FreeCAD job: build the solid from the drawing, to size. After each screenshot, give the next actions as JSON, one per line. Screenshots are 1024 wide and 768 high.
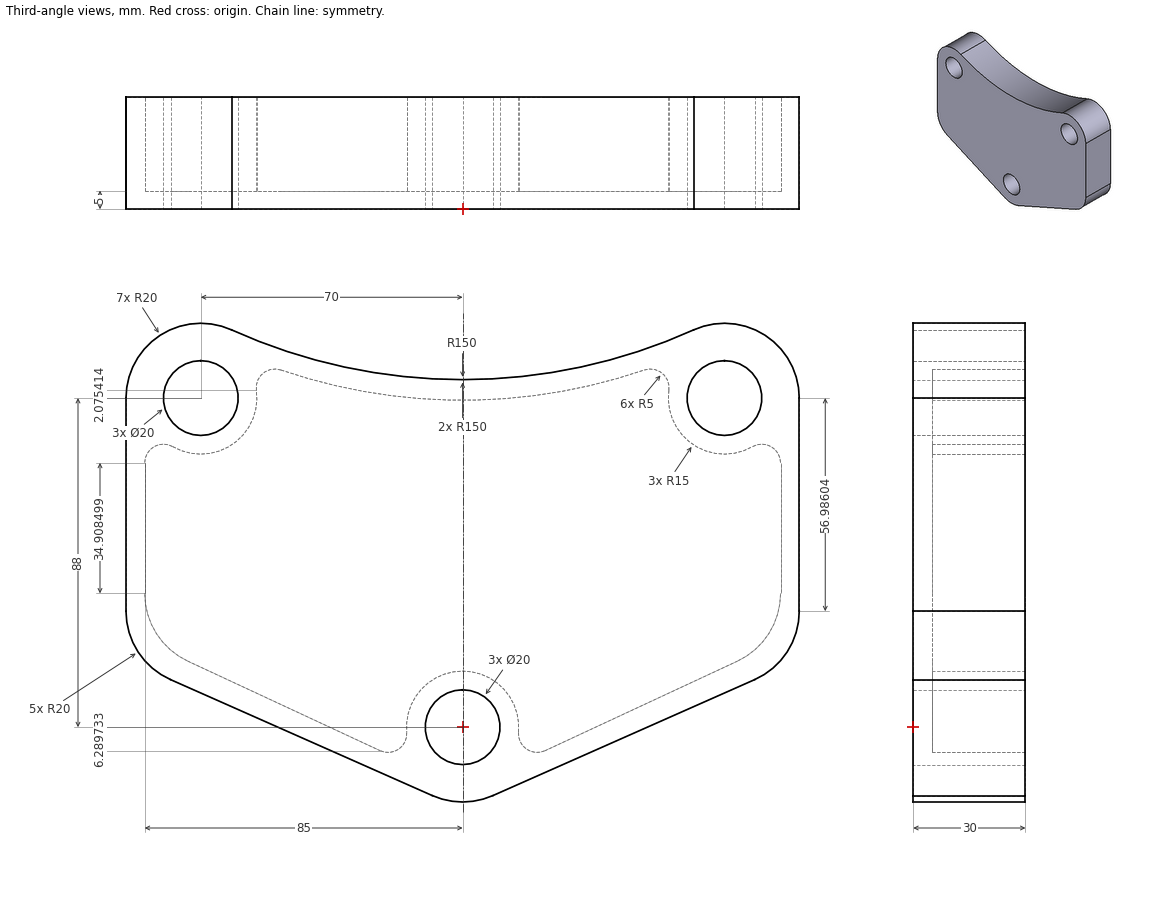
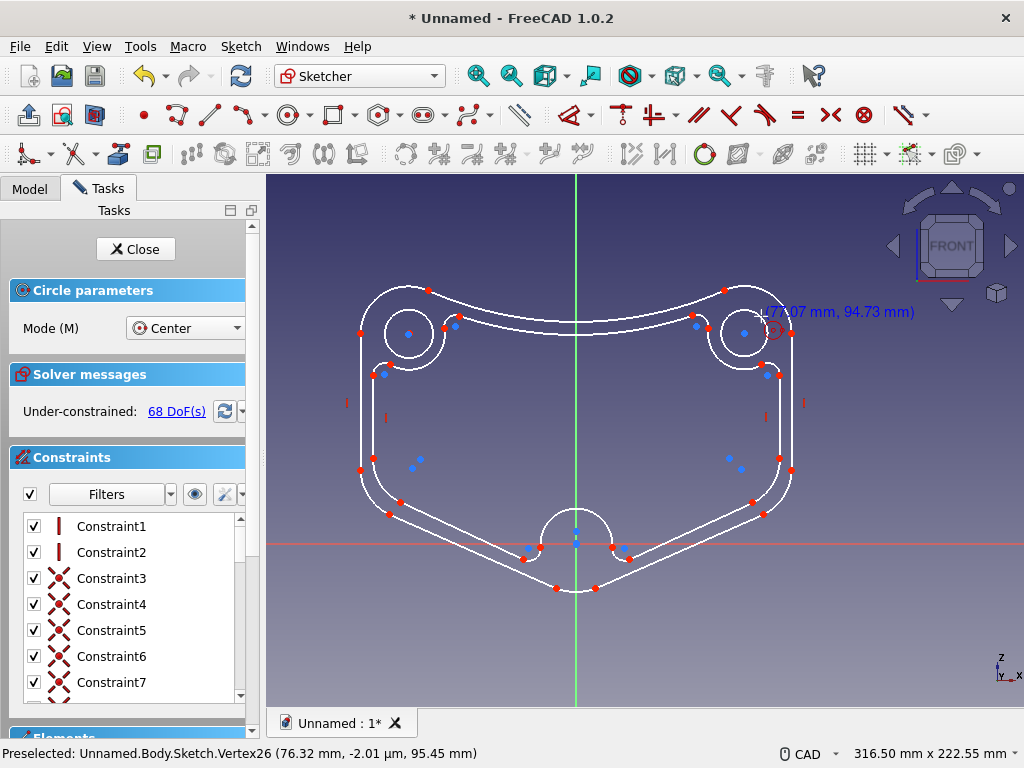
{"action": "left_click", "coordinate": [576, 544]}
{"action": "left_click", "coordinate": [593, 561]}
{"action": "key", "text": "Escape"}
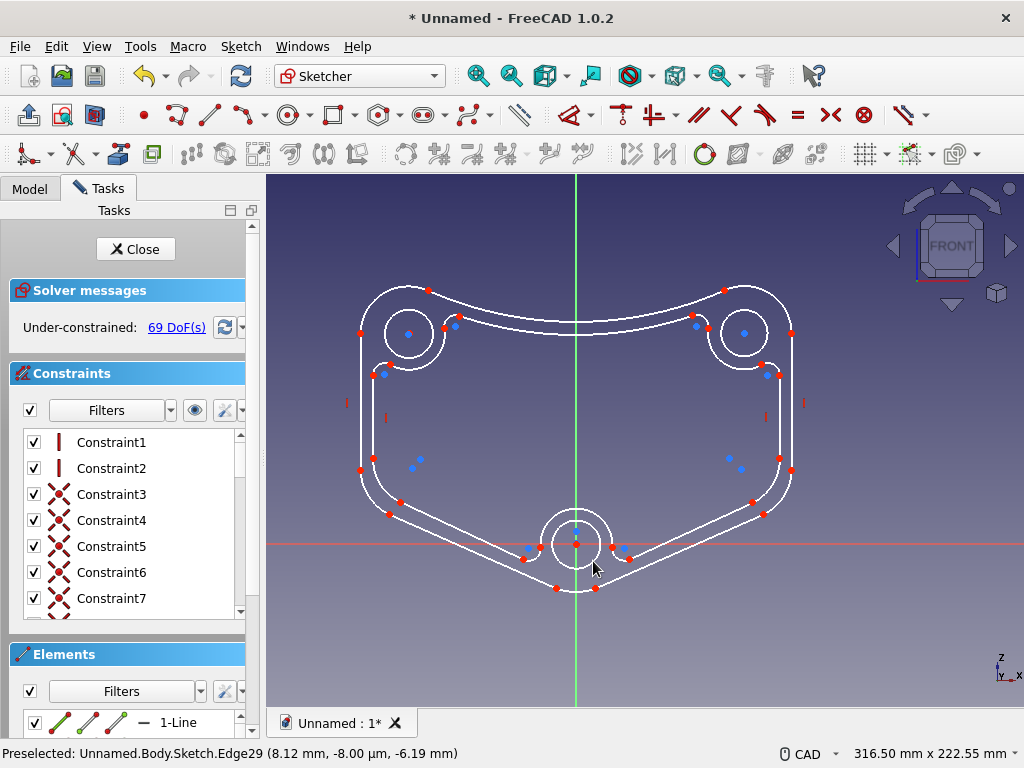
{"action": "left_click", "coordinate": [792, 375]}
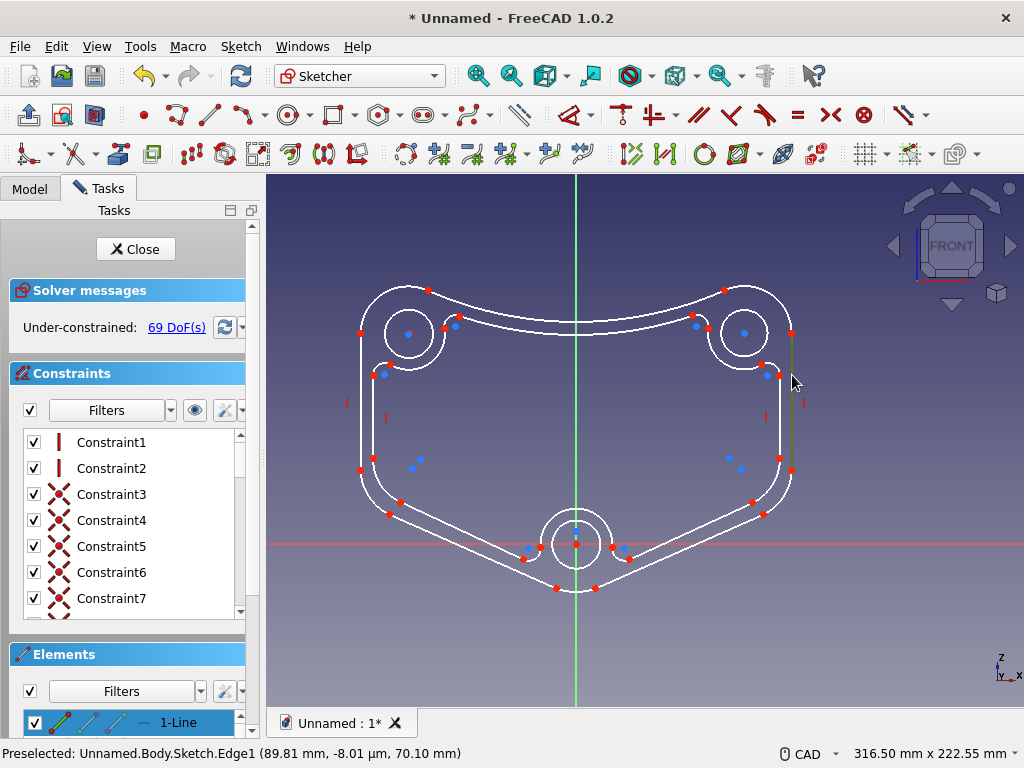
{"action": "left_click", "coordinate": [777, 505]}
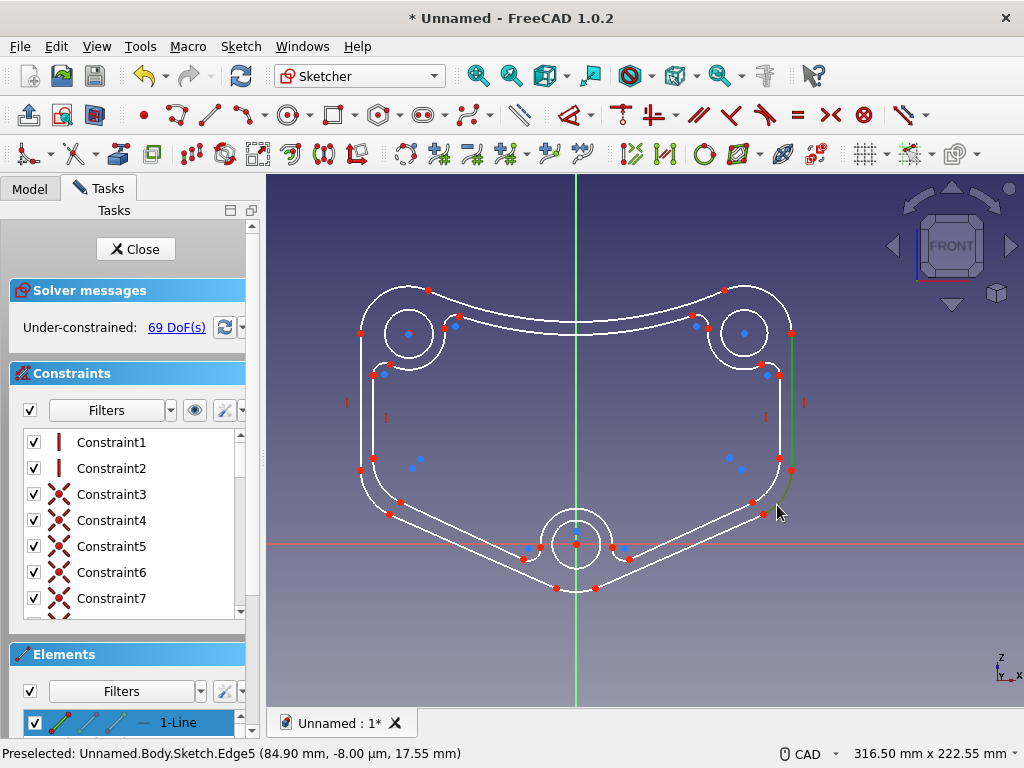
{"action": "key", "text": "t"}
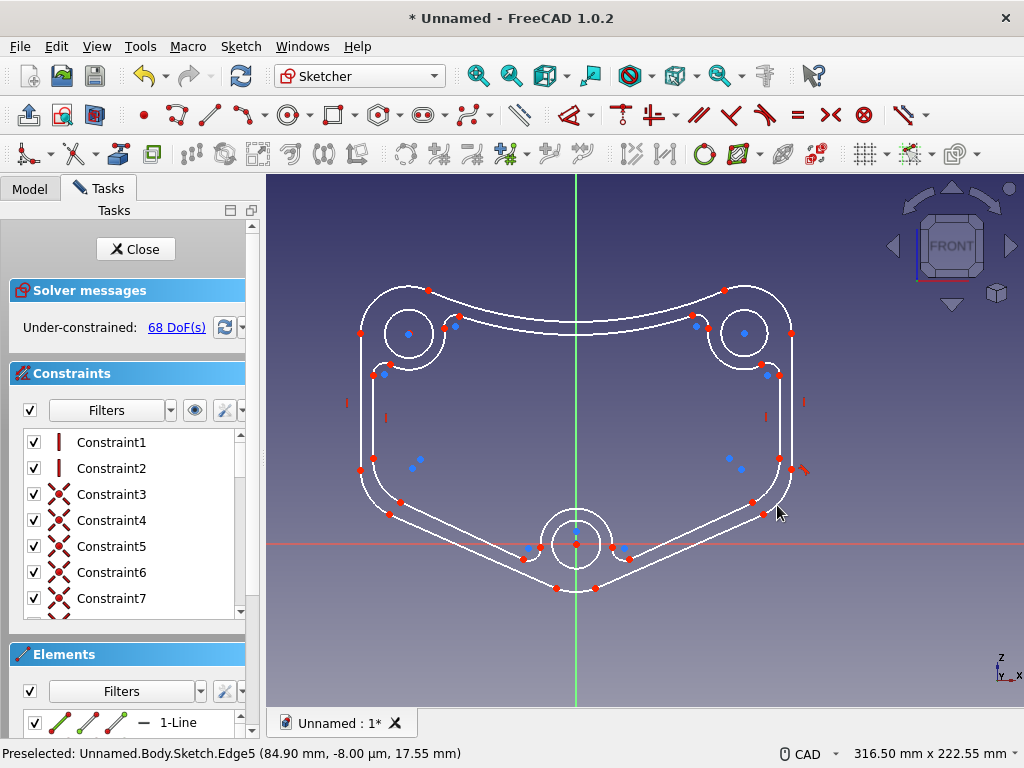
{"action": "left_click", "coordinate": [792, 374]}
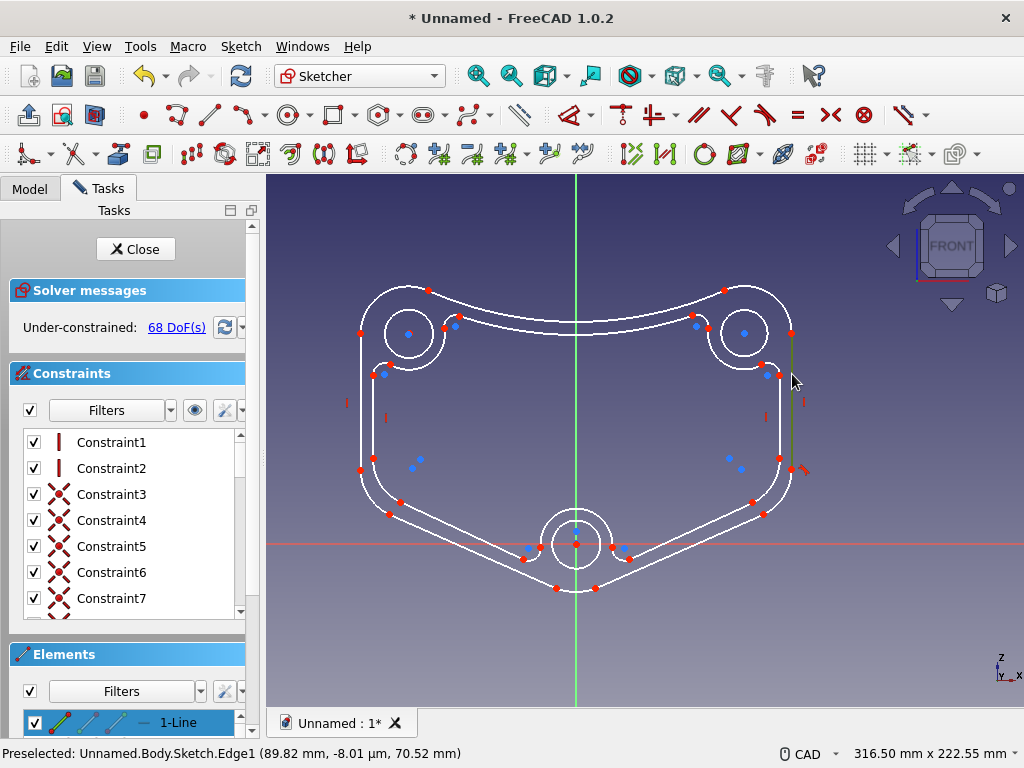
{"action": "left_click", "coordinate": [783, 307]}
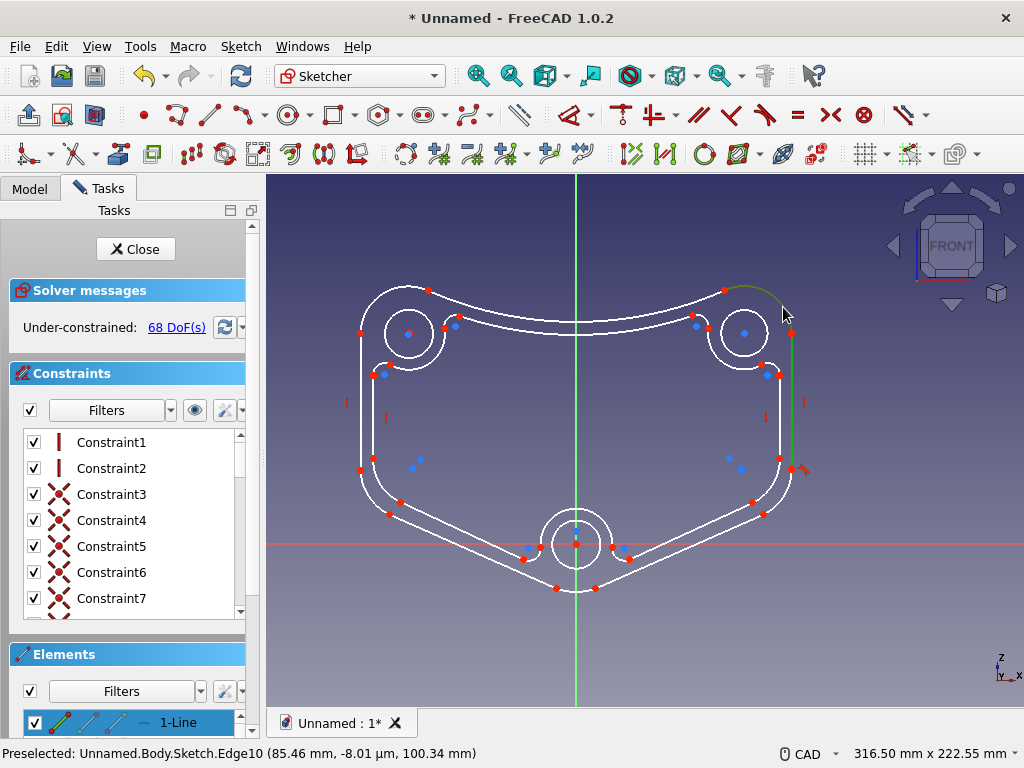
{"action": "left_click", "coordinate": [765, 116]}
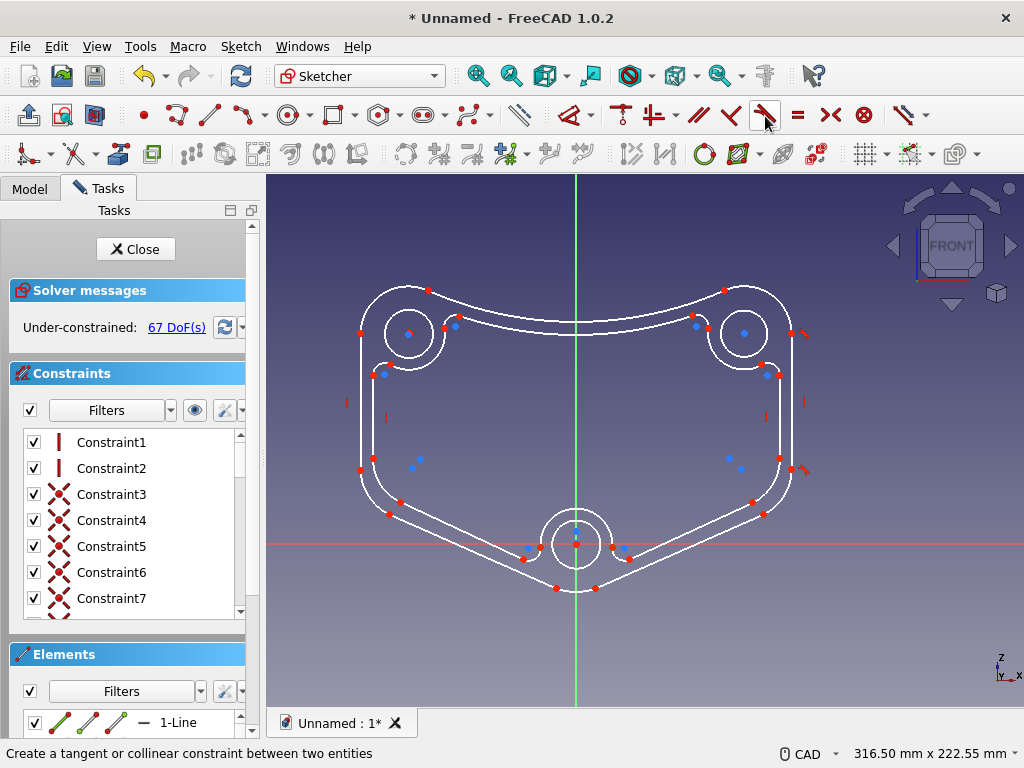
{"action": "left_click", "coordinate": [646, 566]}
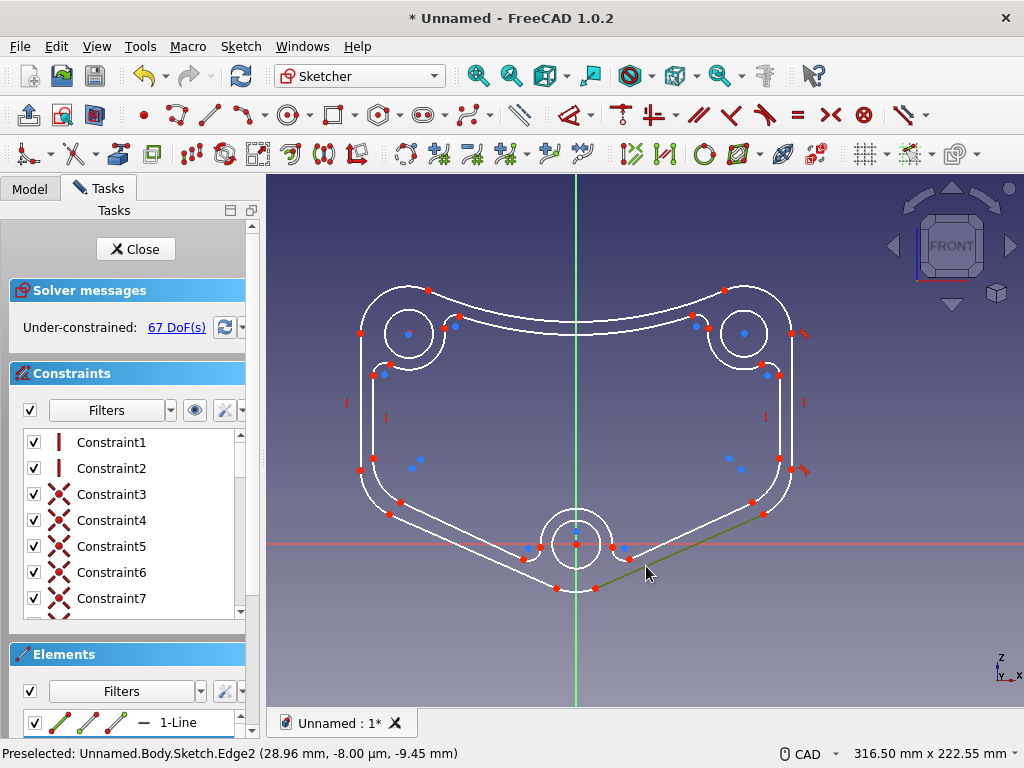
{"action": "left_click", "coordinate": [777, 505]}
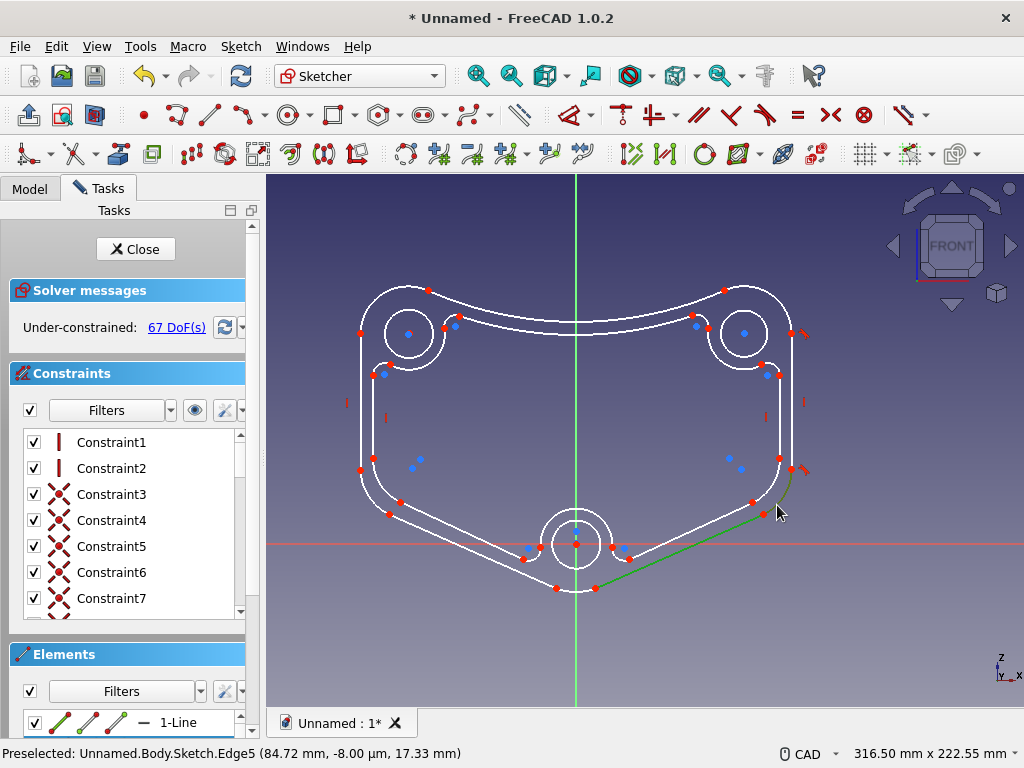
{"action": "left_click", "coordinate": [765, 116]}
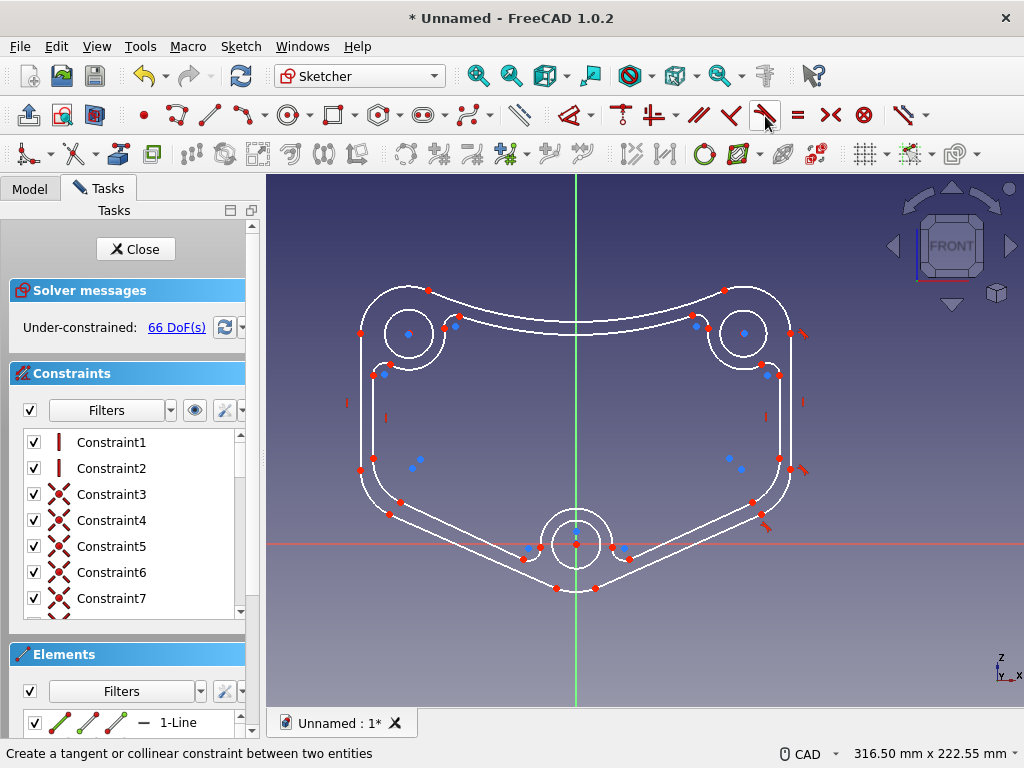
{"action": "left_click", "coordinate": [645, 566]}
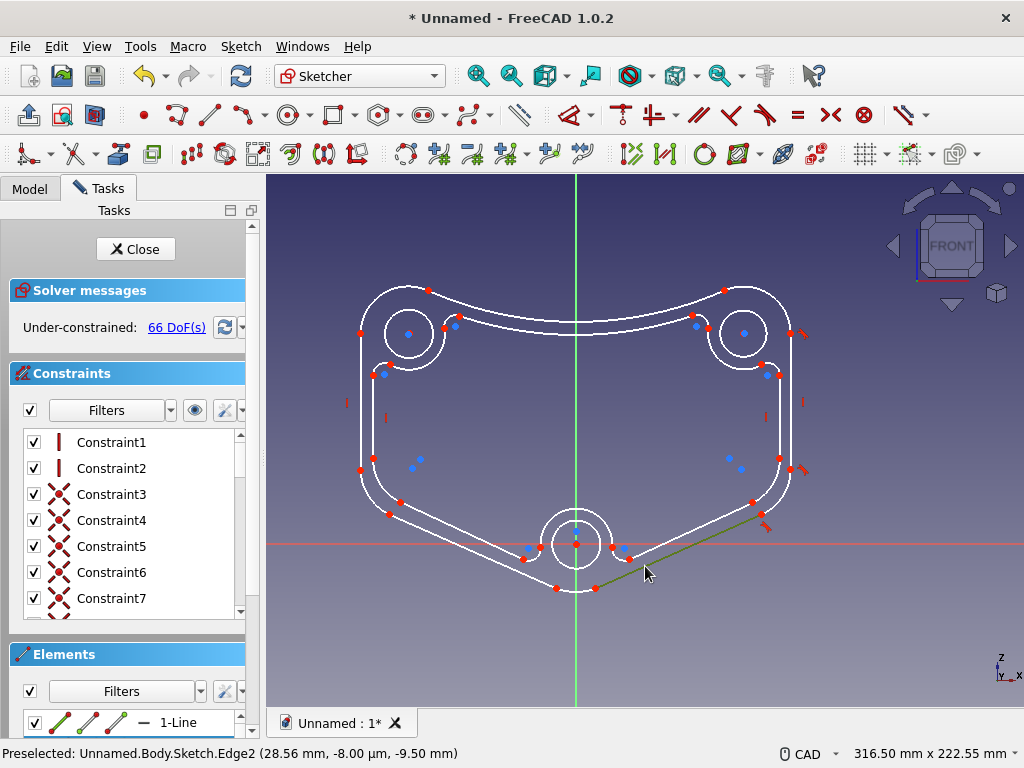
{"action": "left_click", "coordinate": [576, 592]}